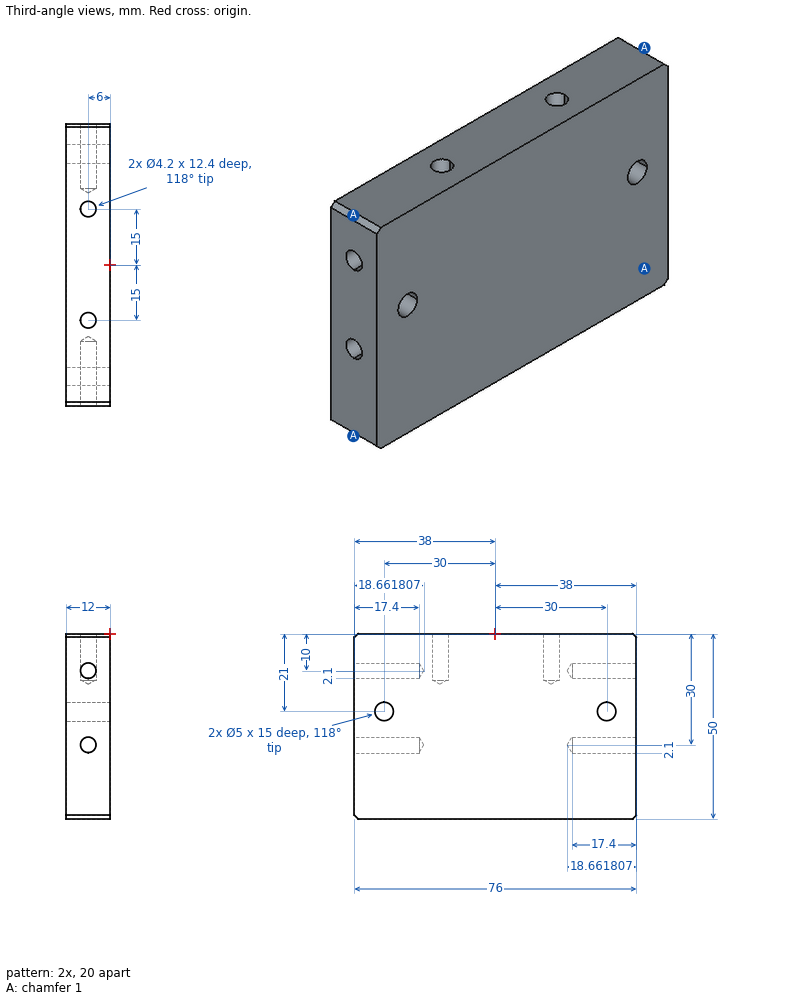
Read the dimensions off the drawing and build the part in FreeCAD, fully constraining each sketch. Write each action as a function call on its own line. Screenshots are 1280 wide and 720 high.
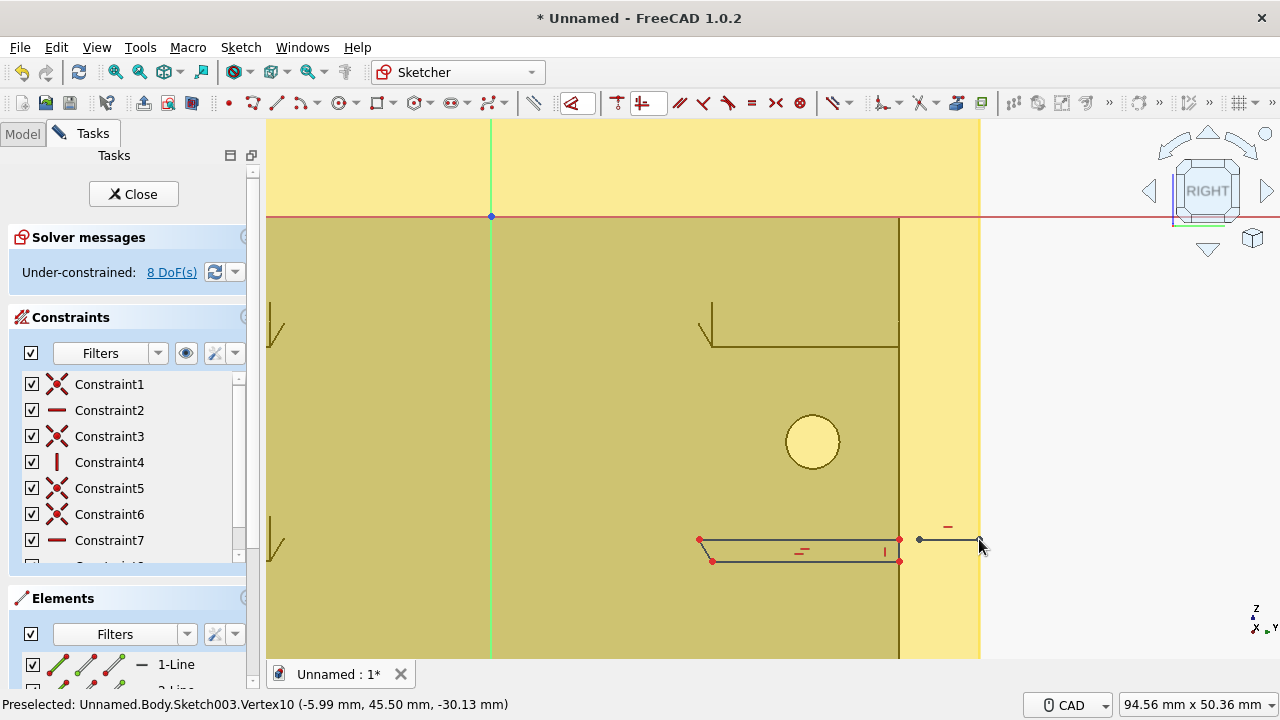
click(937, 540)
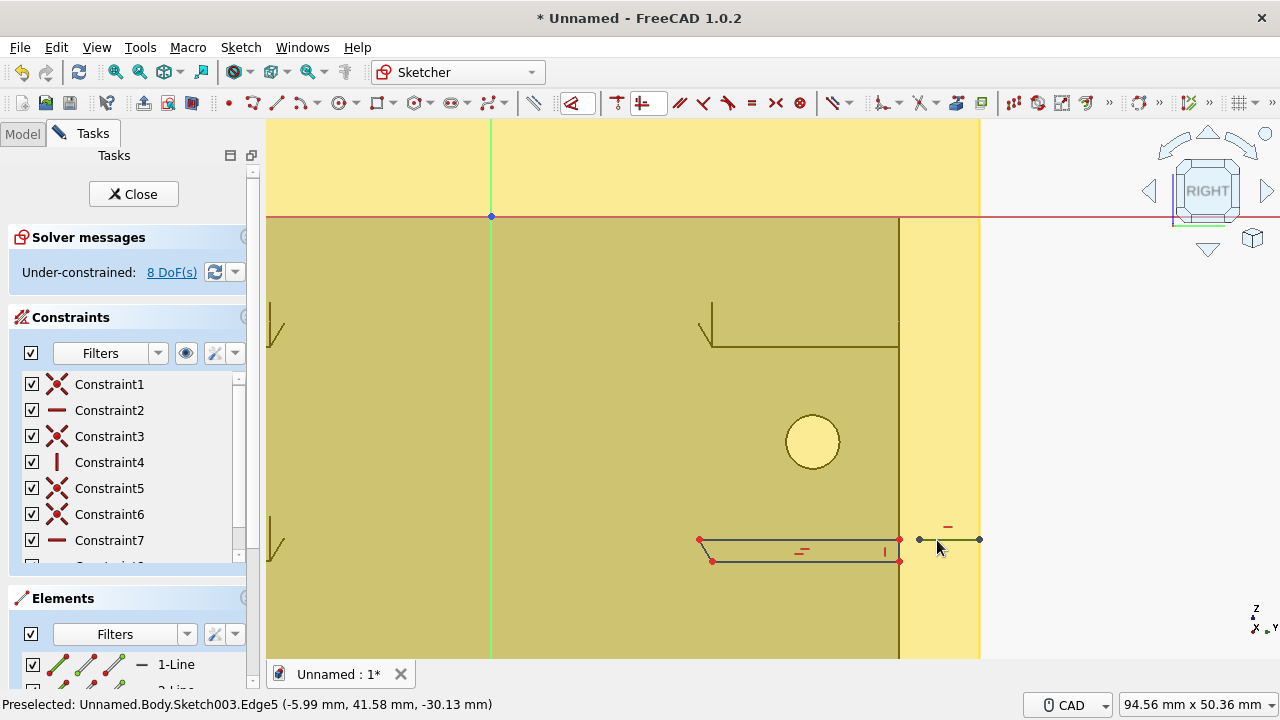
key(g)
key(n)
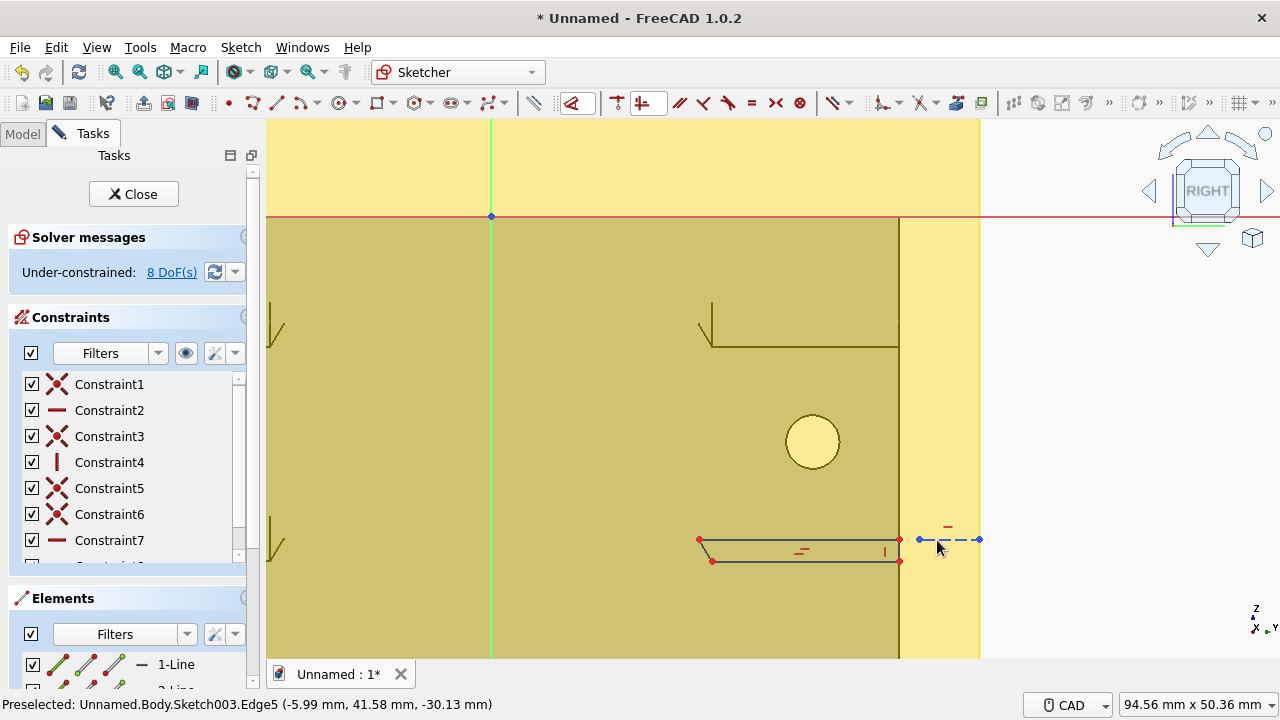
scroll(899, 551, up, 3)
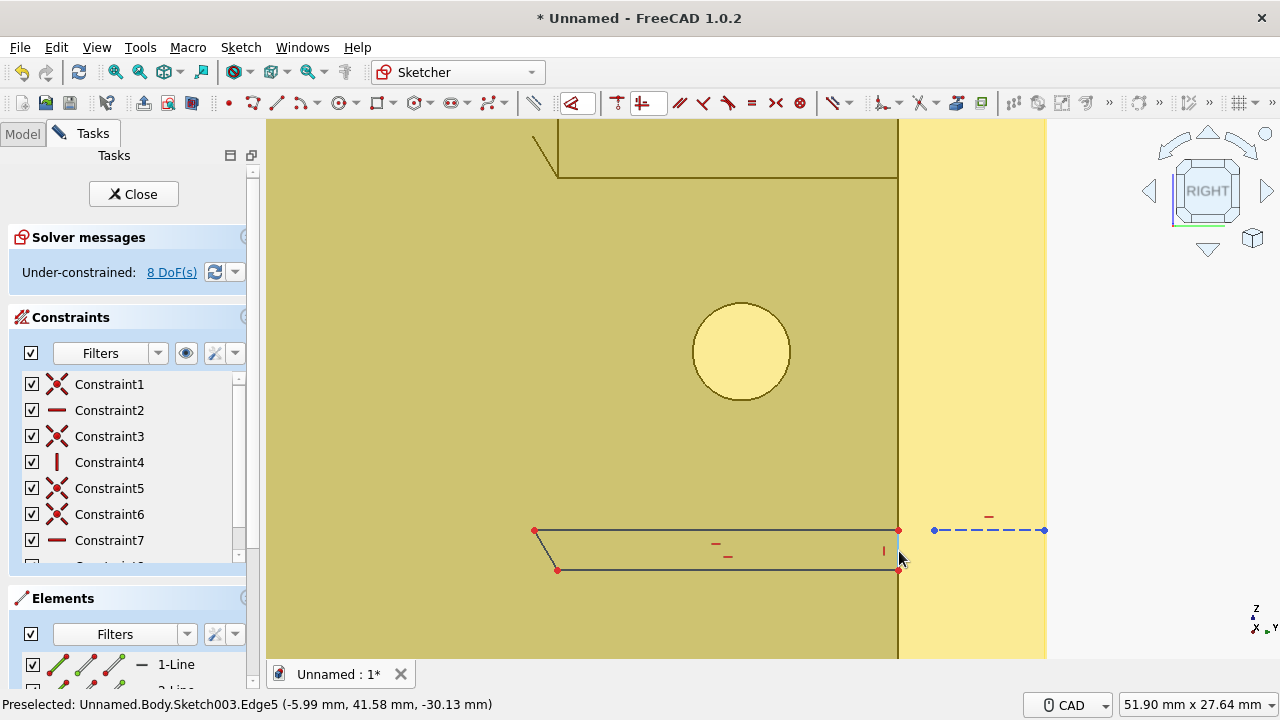
click(898, 550)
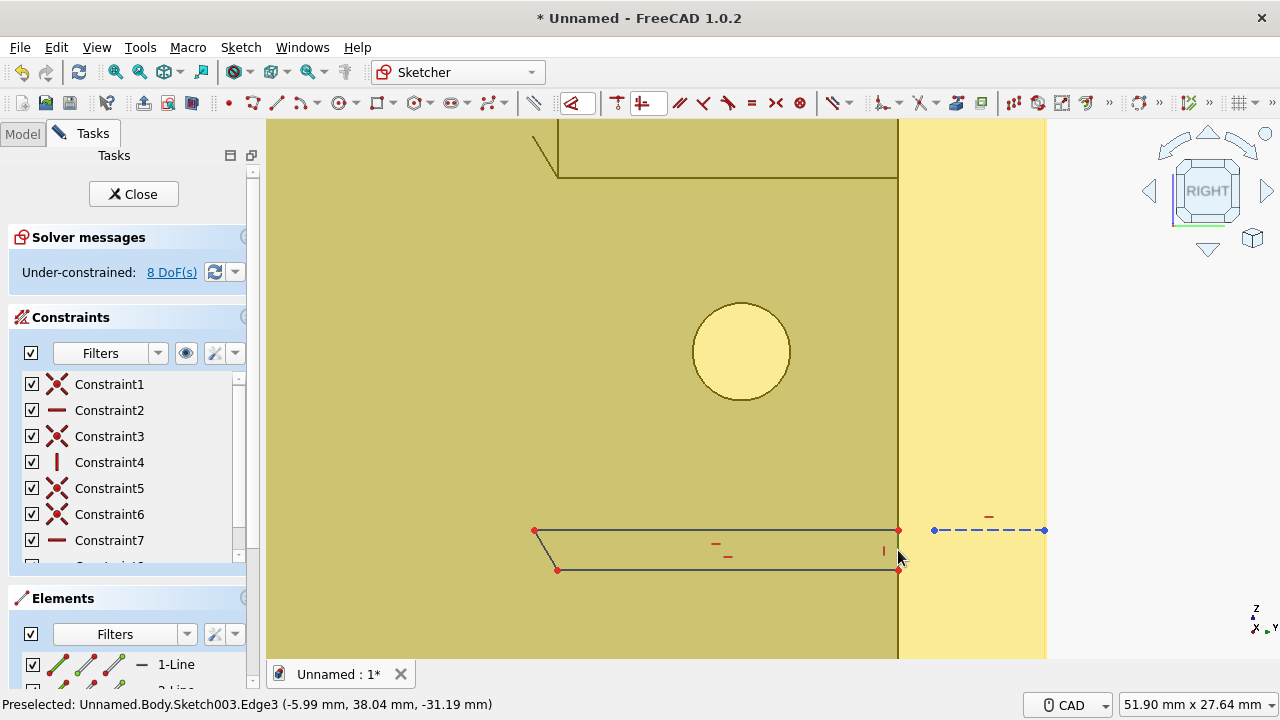
click(590, 104)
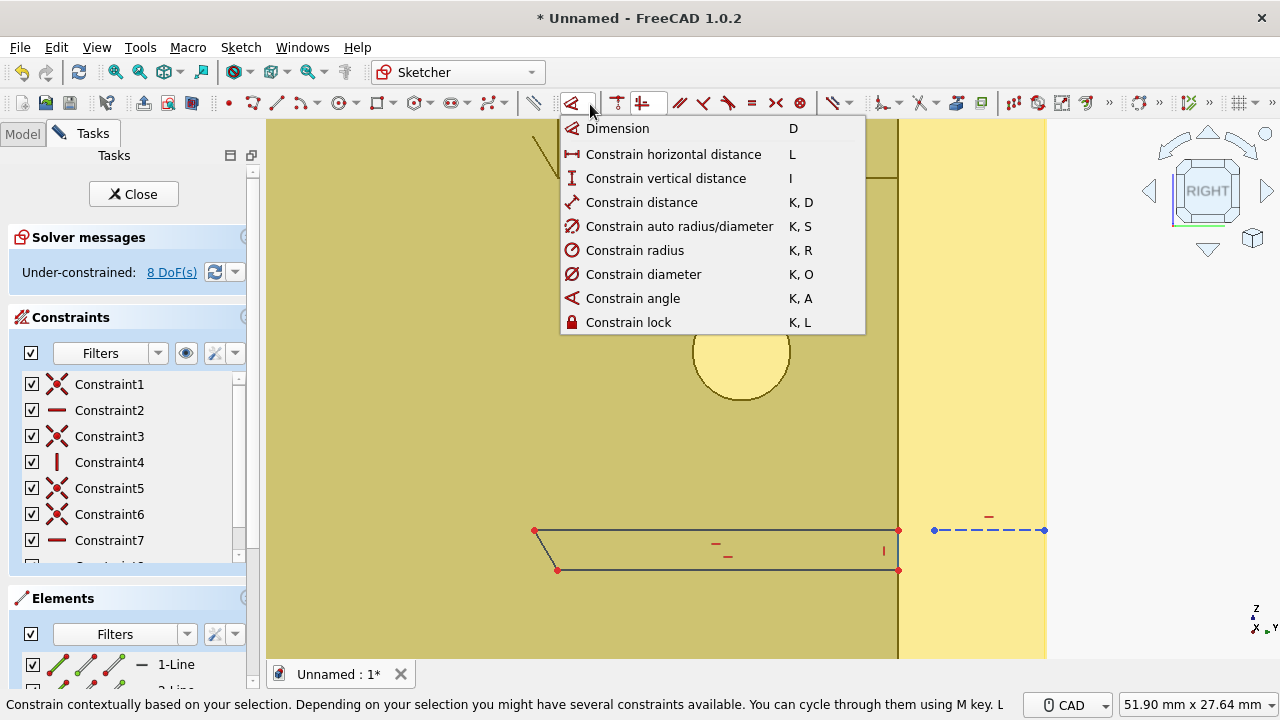
click(713, 178)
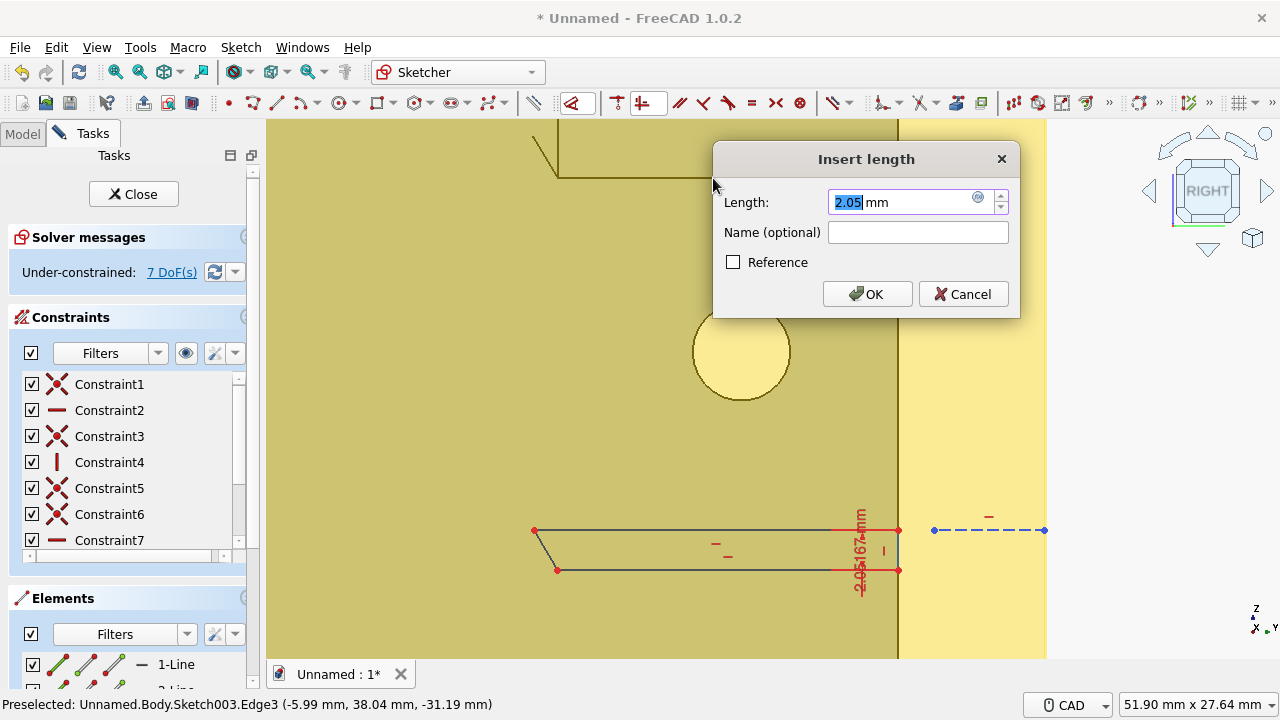
text(2.1)
key(Return)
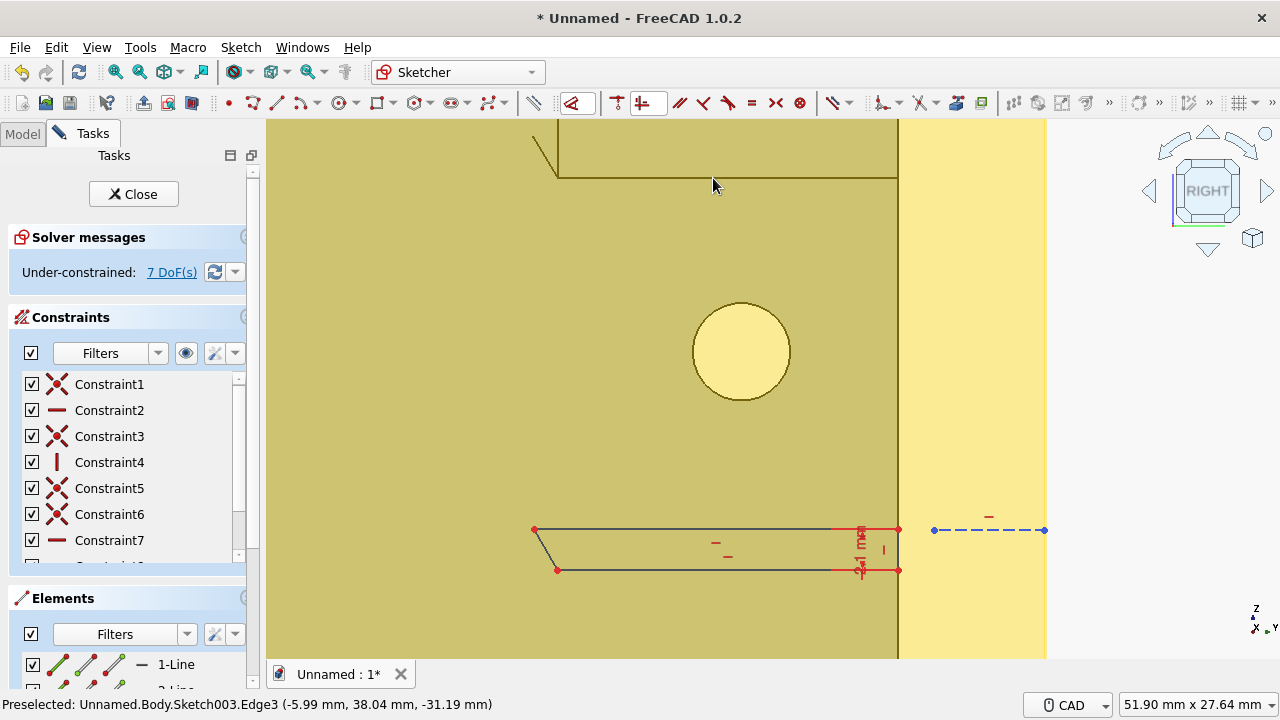
click(534, 529)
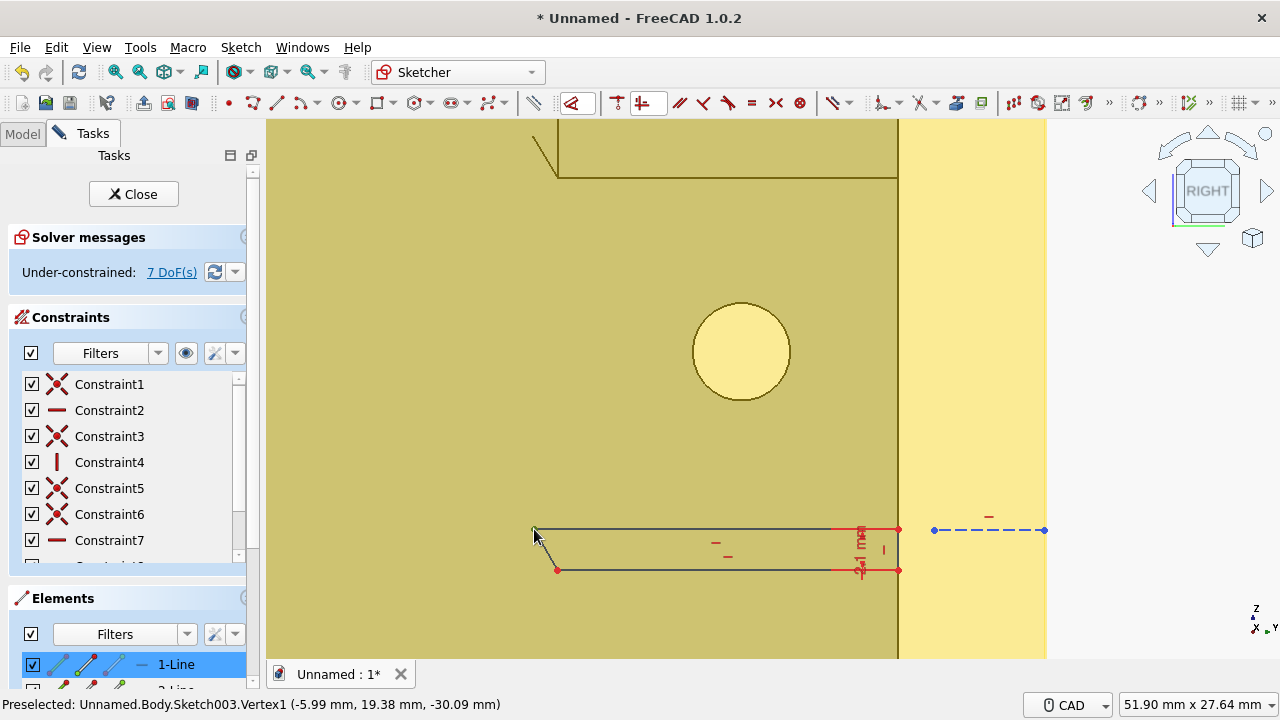
click(590, 104)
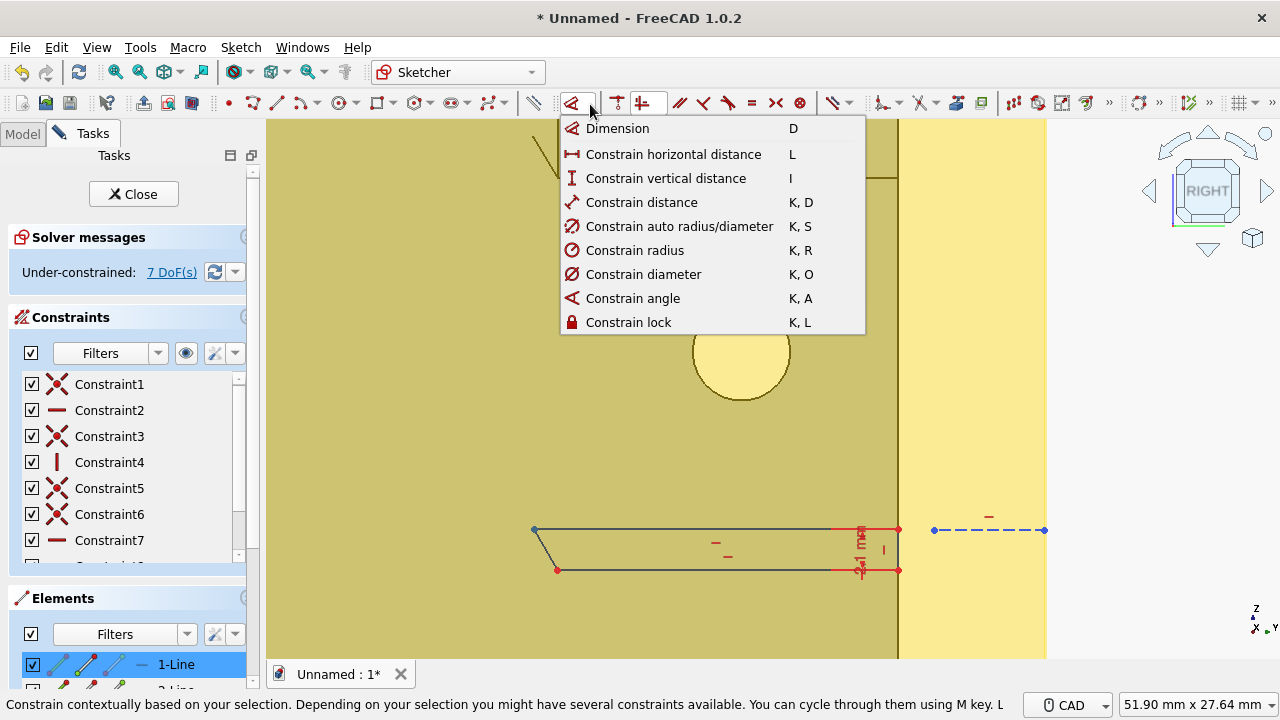
click(713, 178)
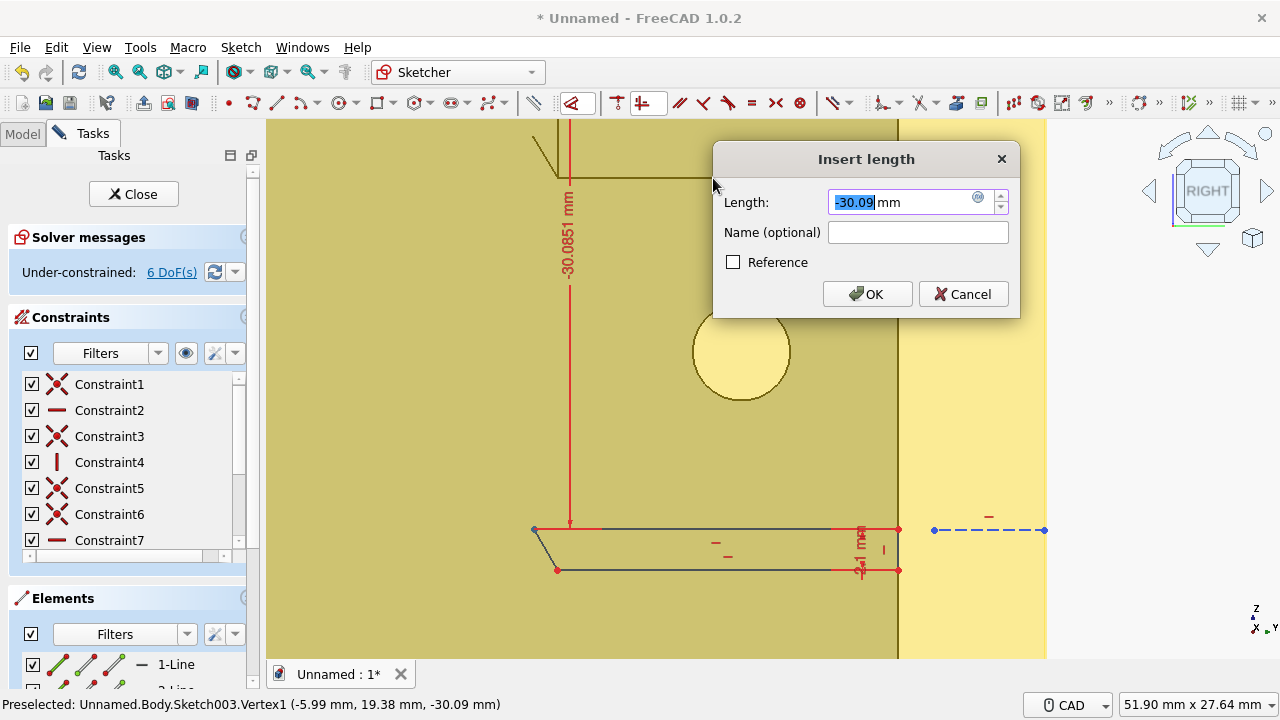
text(-30)
key(Return)